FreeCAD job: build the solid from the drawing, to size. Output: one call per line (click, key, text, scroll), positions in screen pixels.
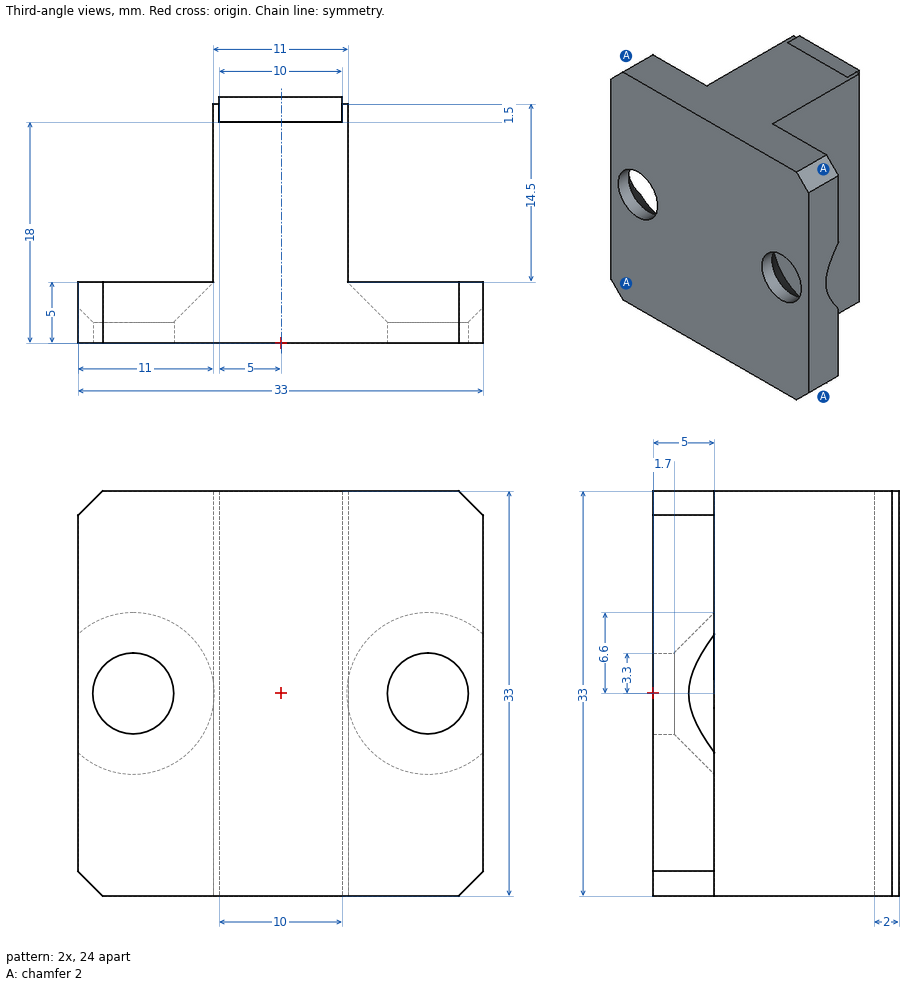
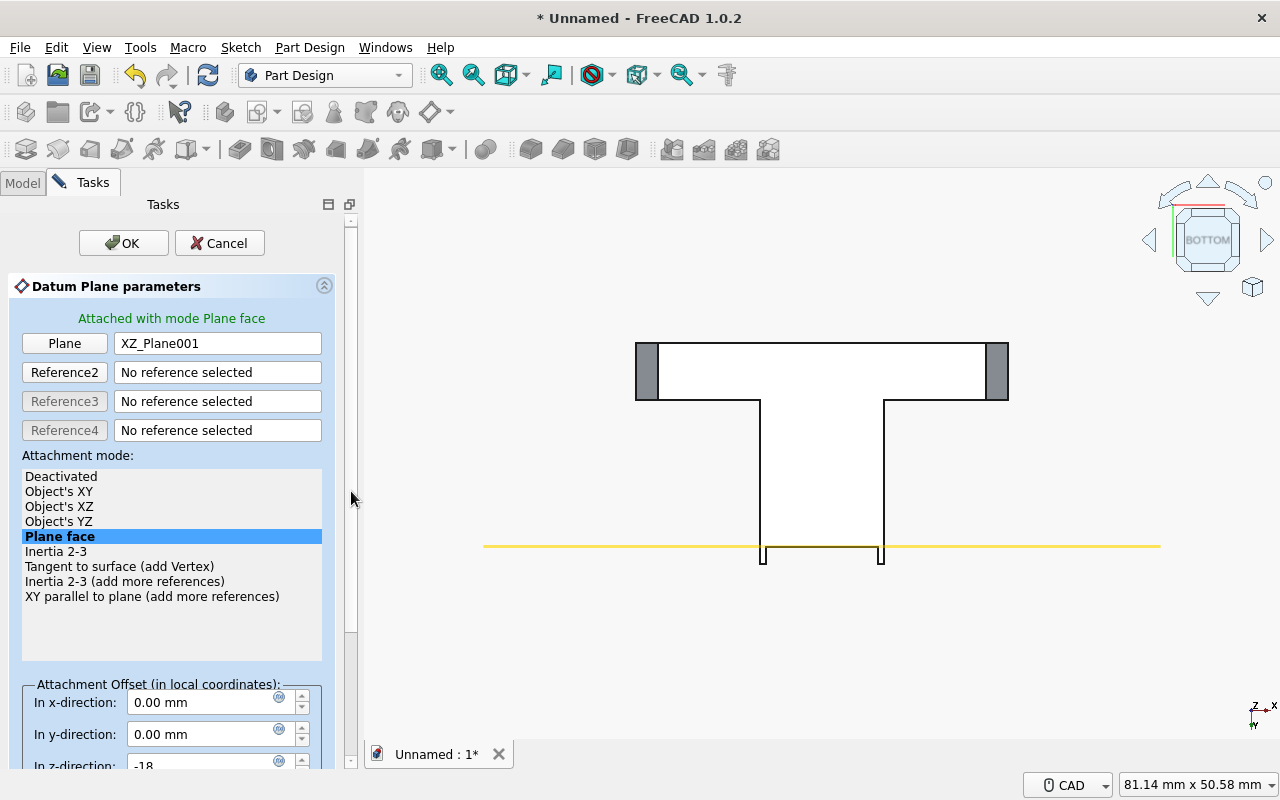
click(124, 243)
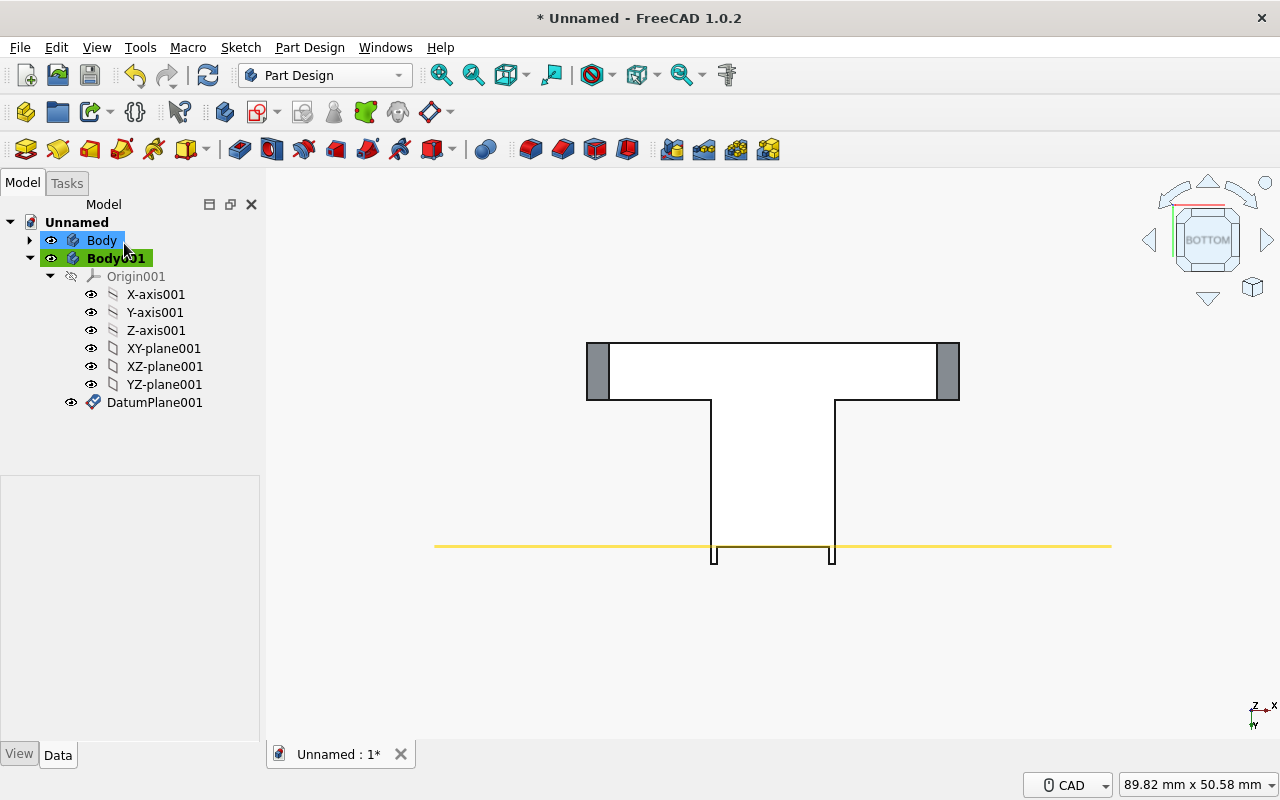
click(116, 402)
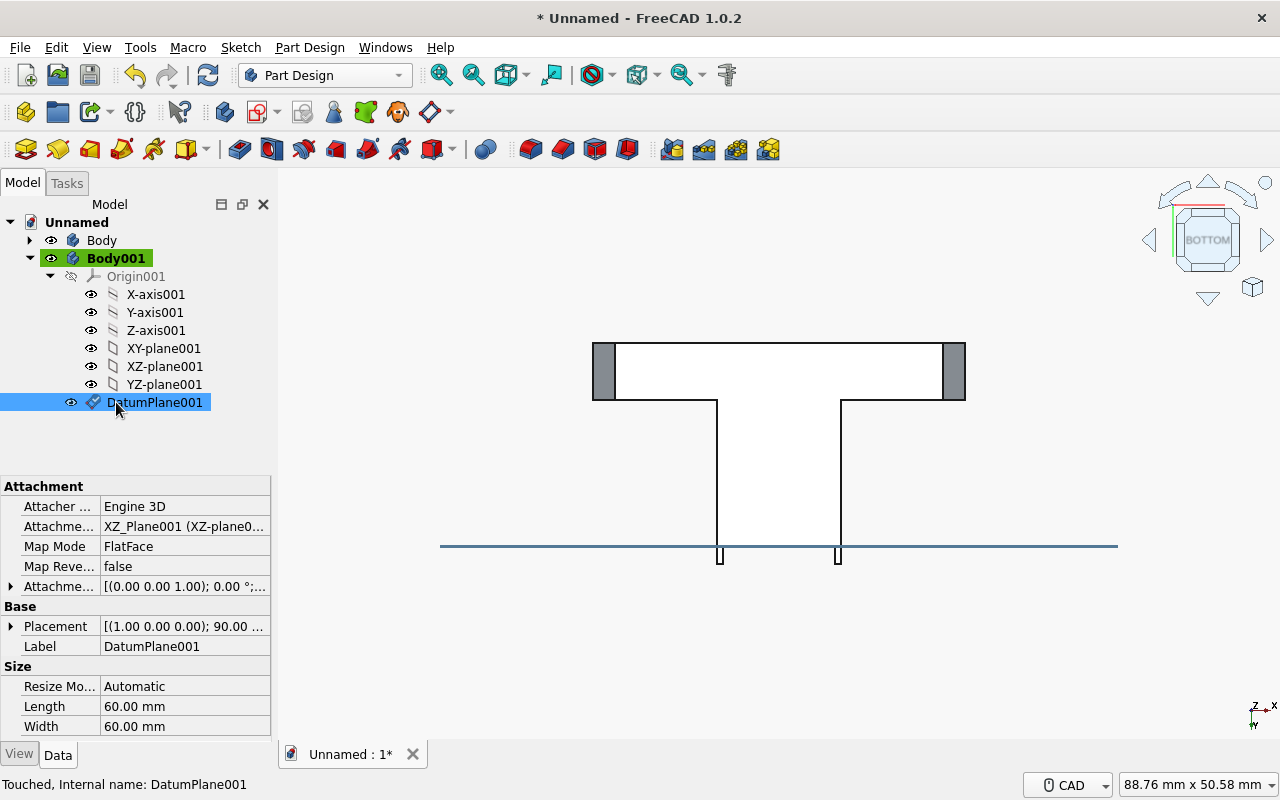
click(258, 112)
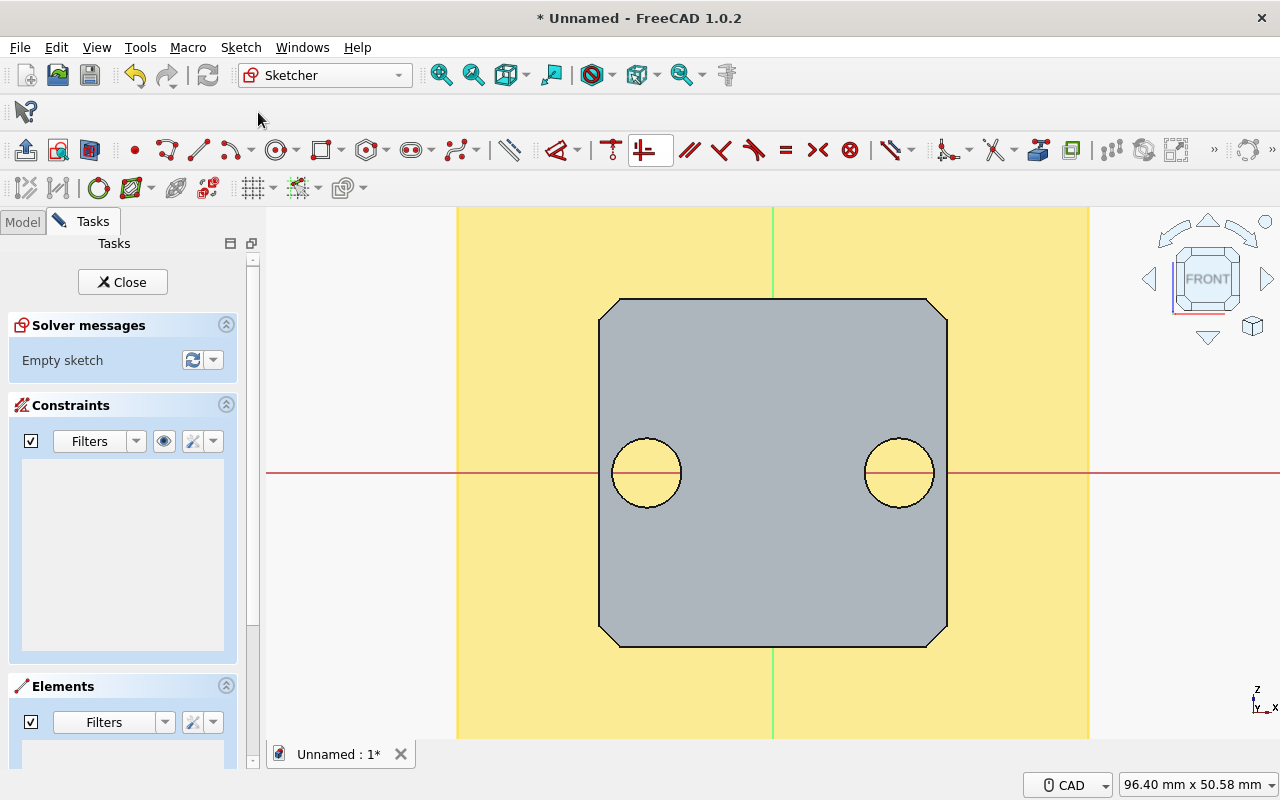
key(g)
key(v)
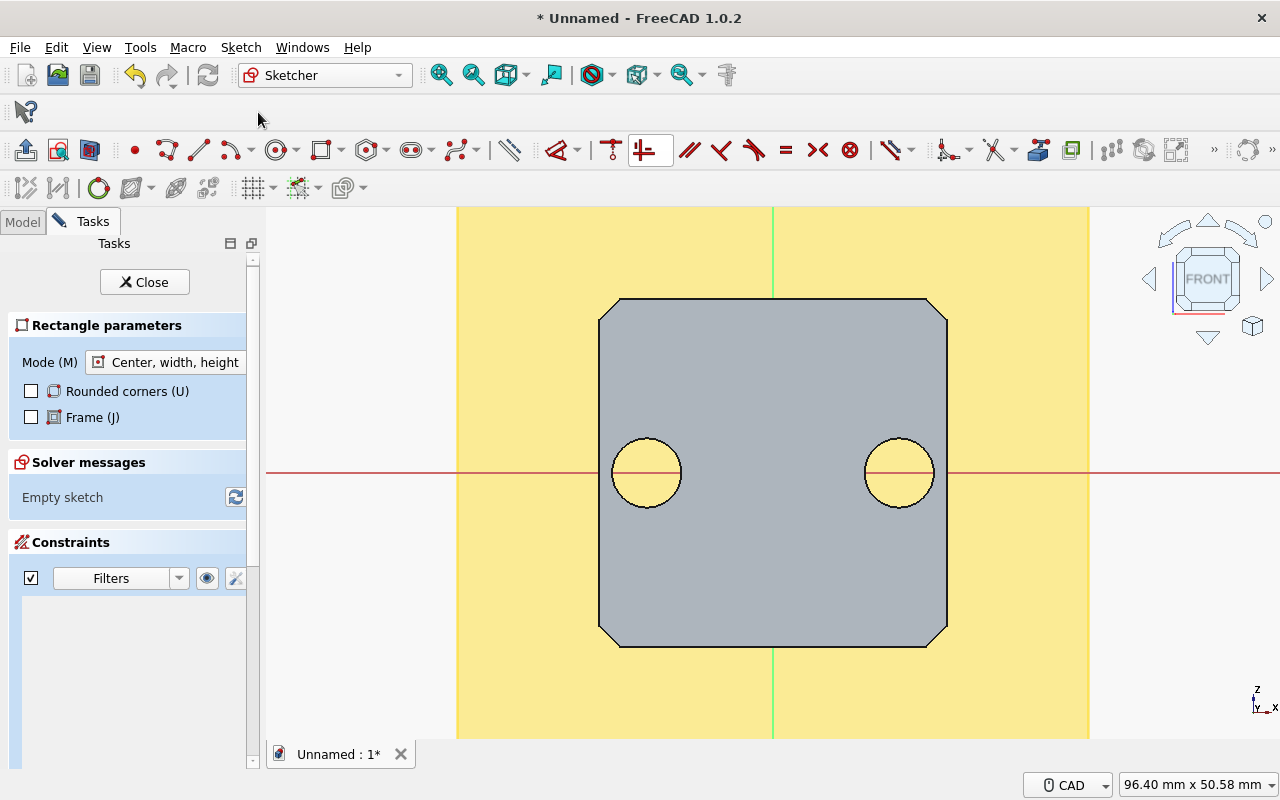
click(773, 473)
move(826, 299)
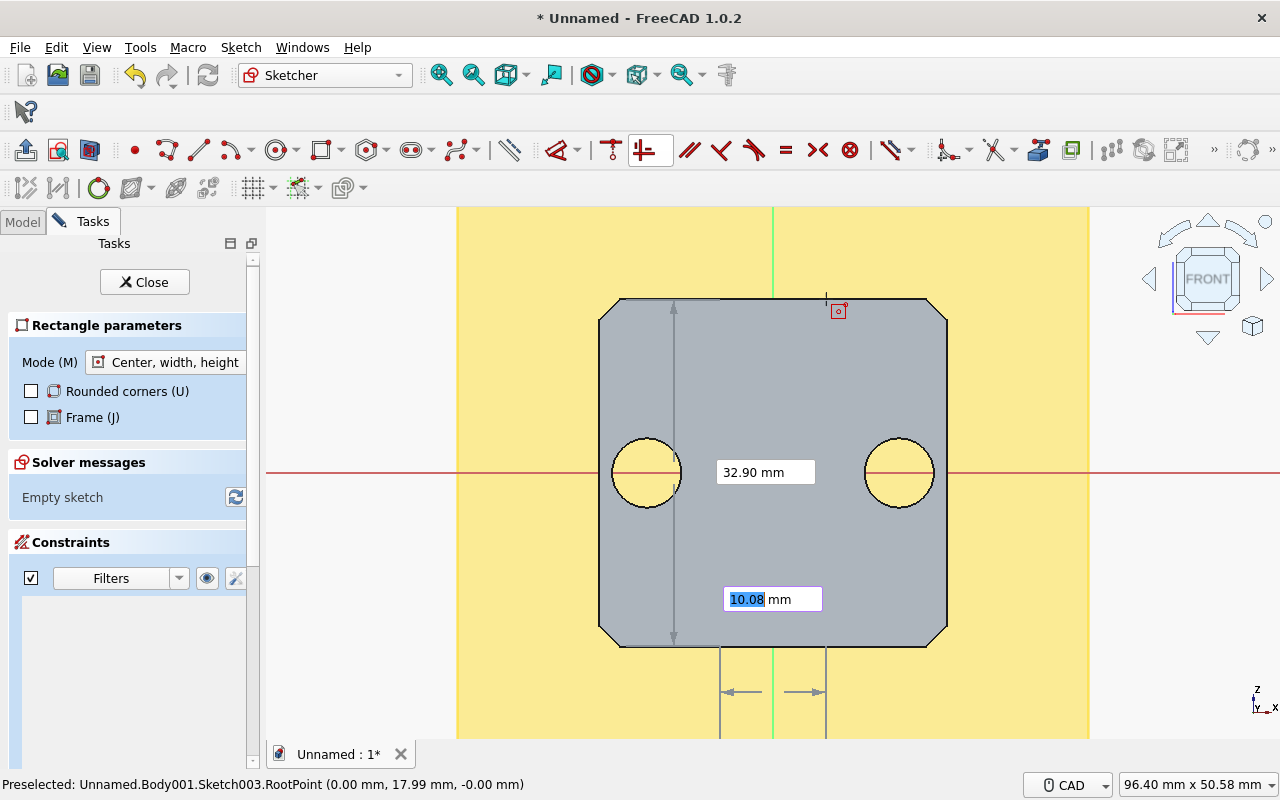
text(10)
key(Tab)
text(33)
key(Return)
key(Escape)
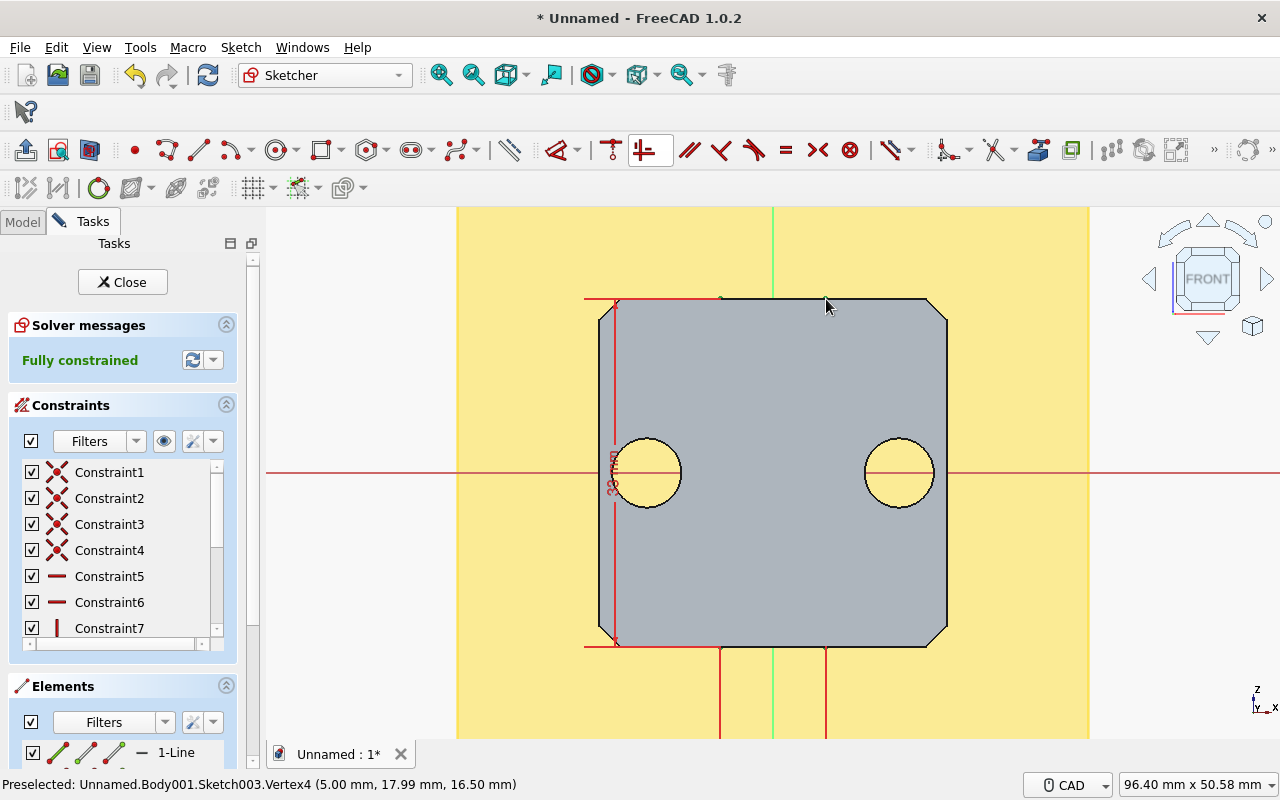
click(123, 282)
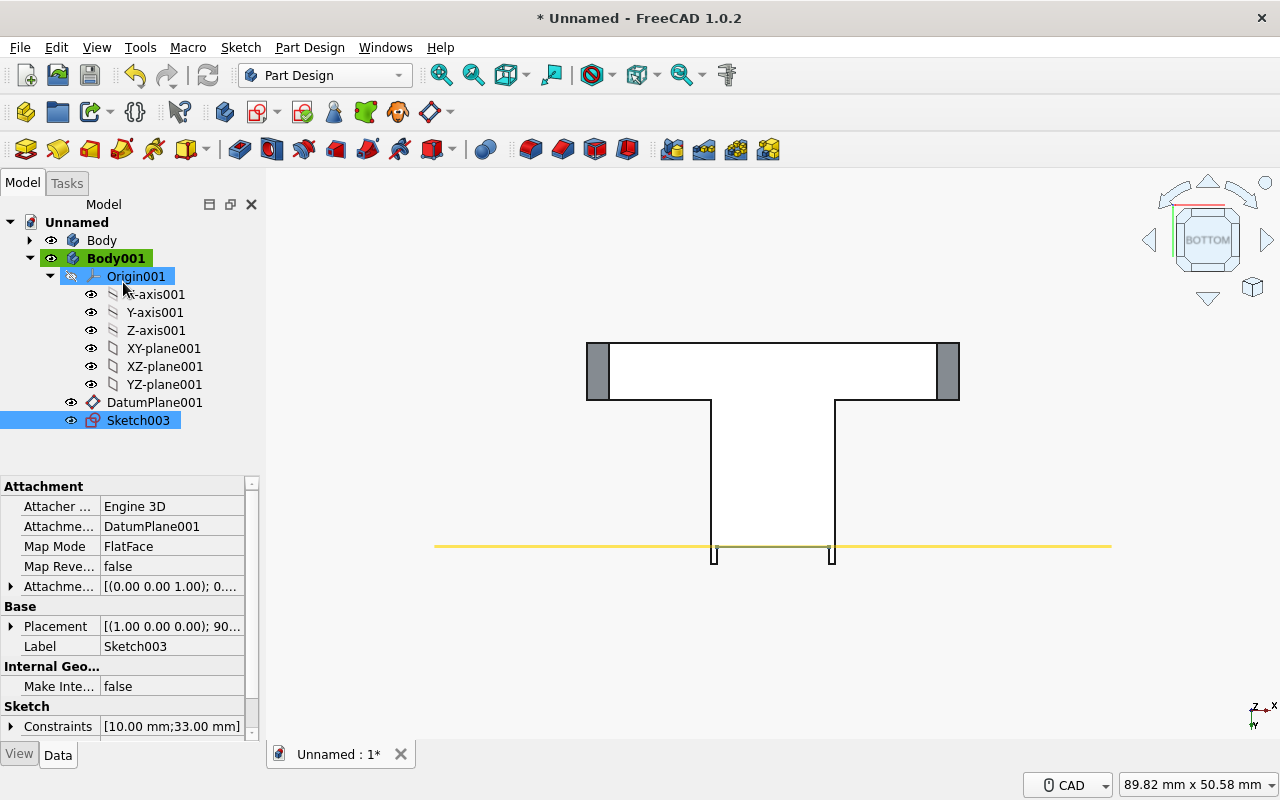
click(26, 150)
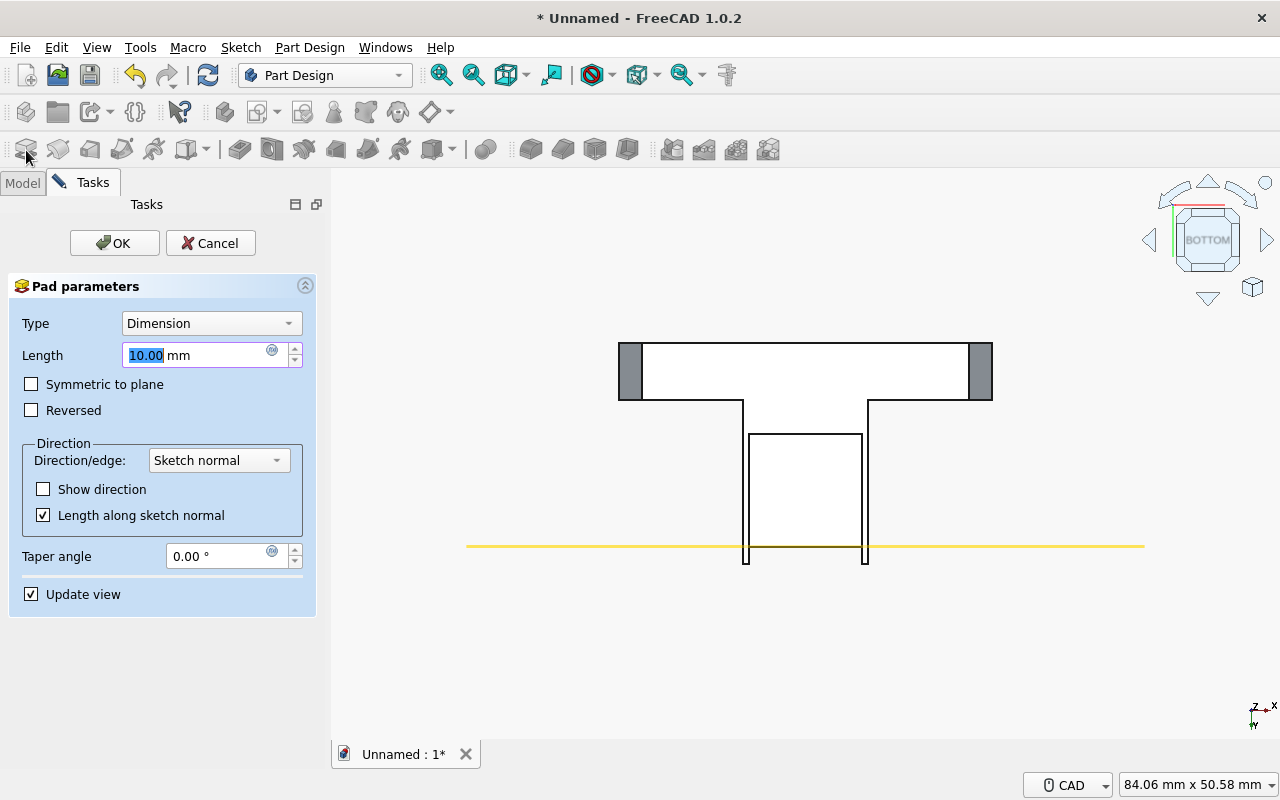
text(2)
key(Tab)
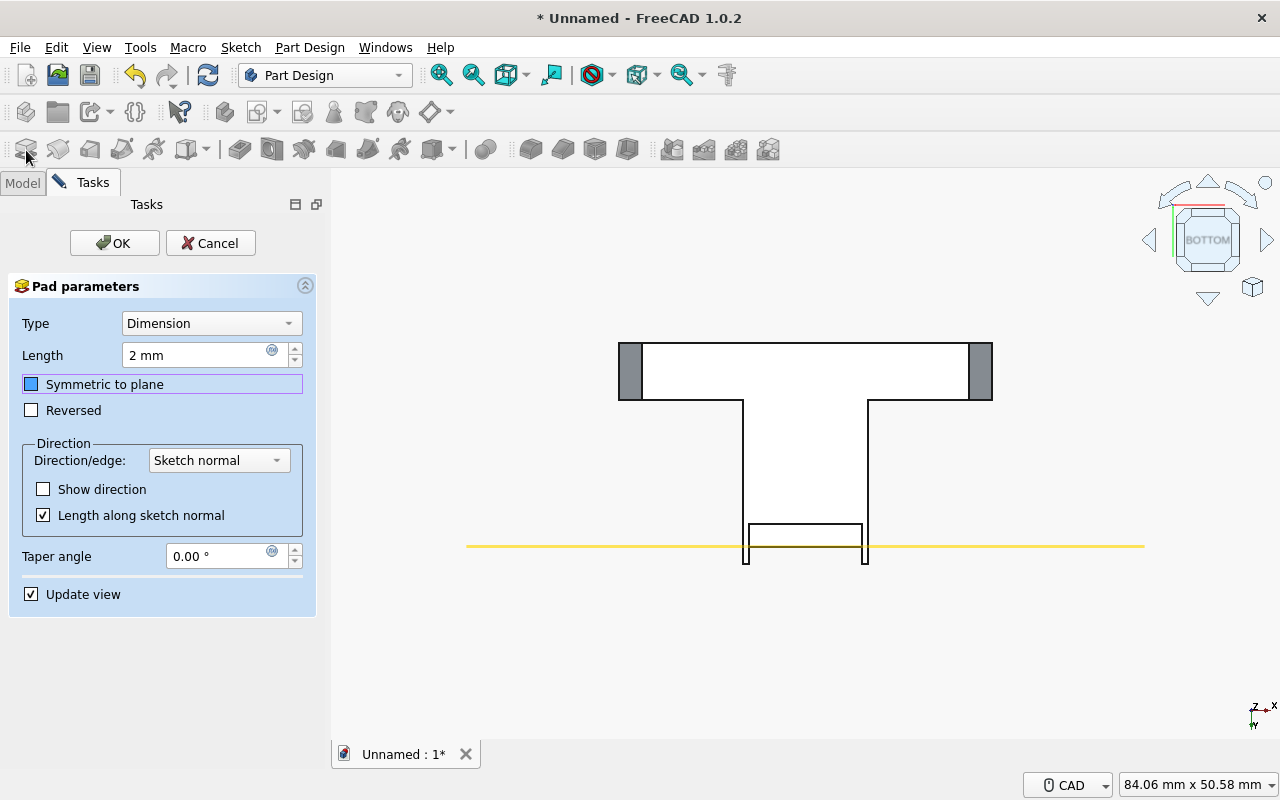
click(30, 410)